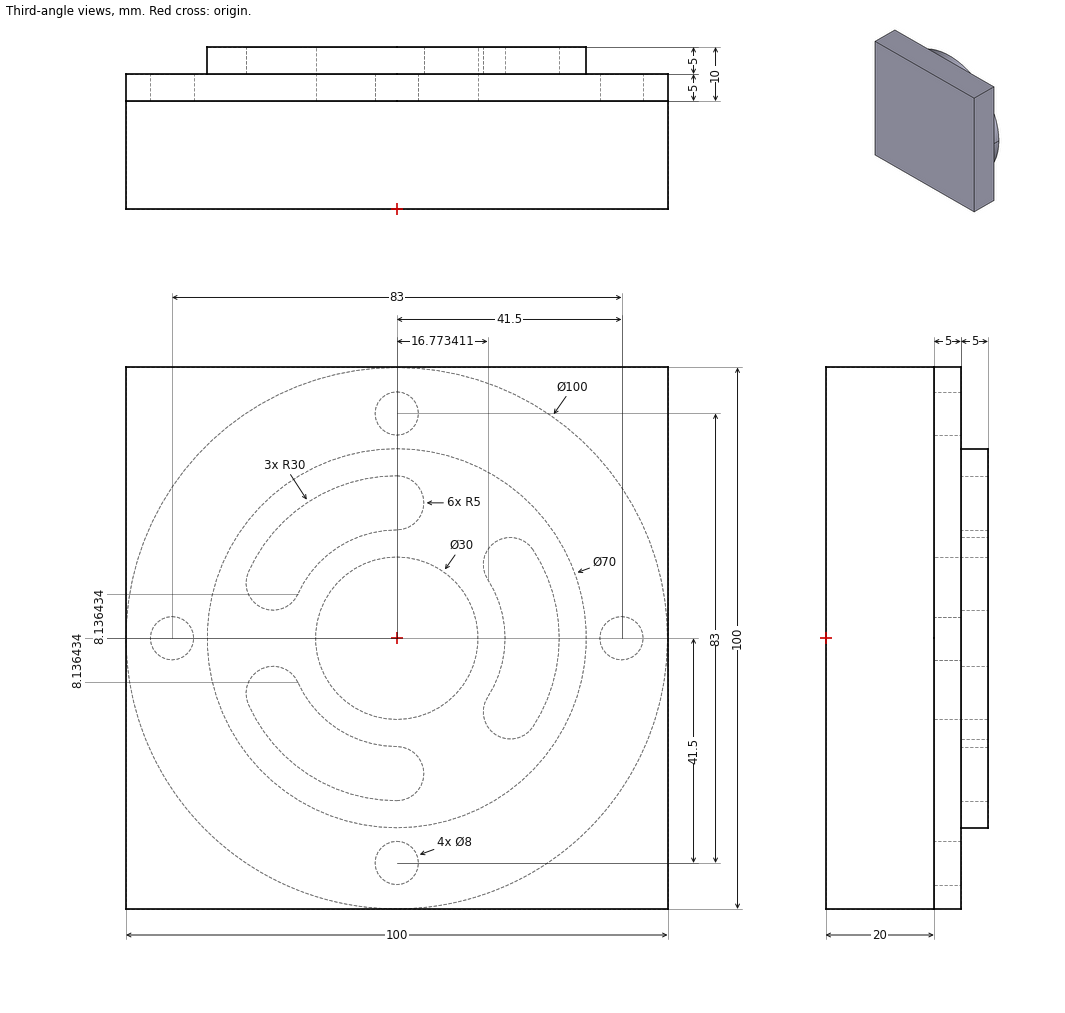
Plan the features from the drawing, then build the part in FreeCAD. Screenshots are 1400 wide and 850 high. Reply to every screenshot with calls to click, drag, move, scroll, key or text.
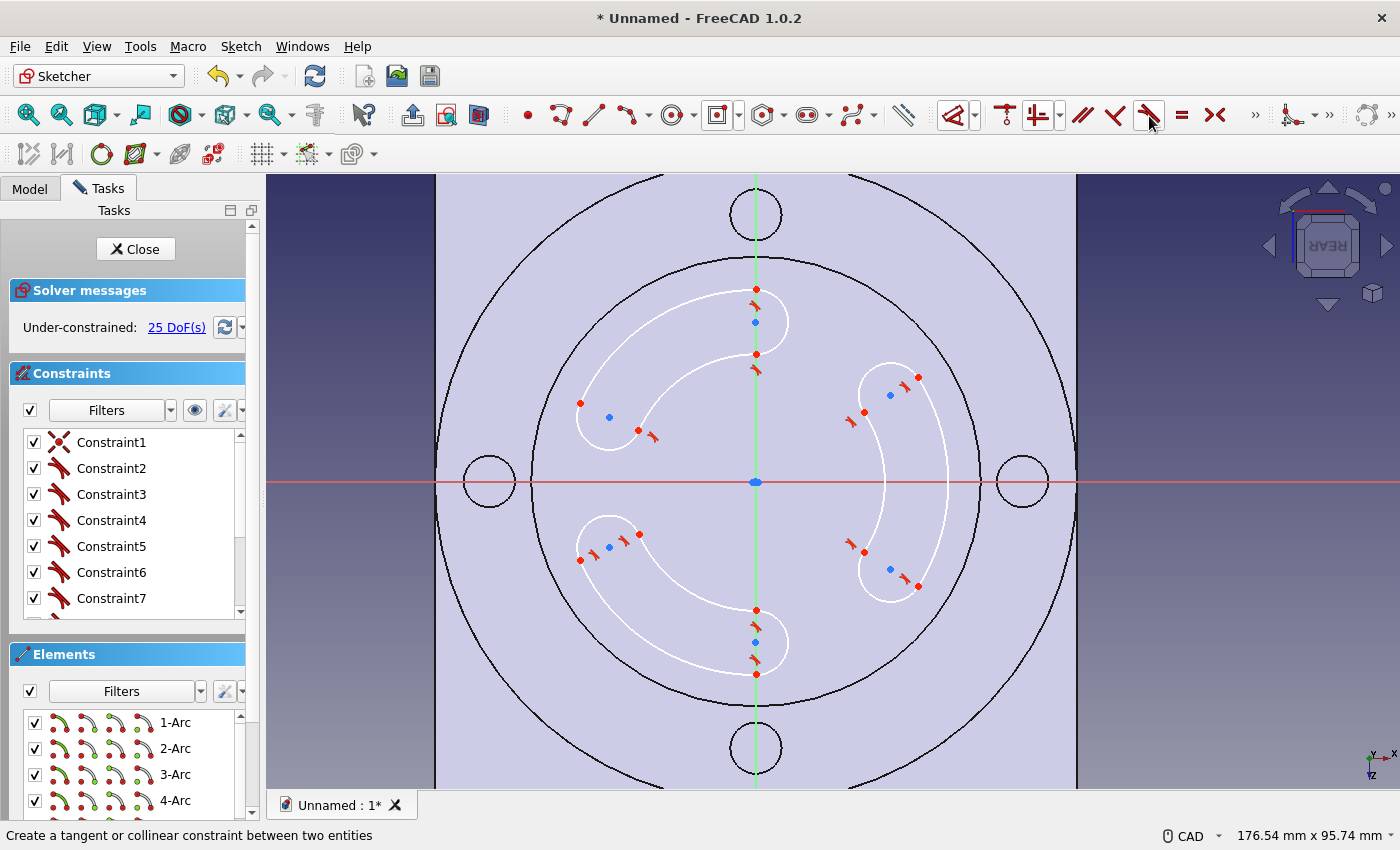
click(691, 301)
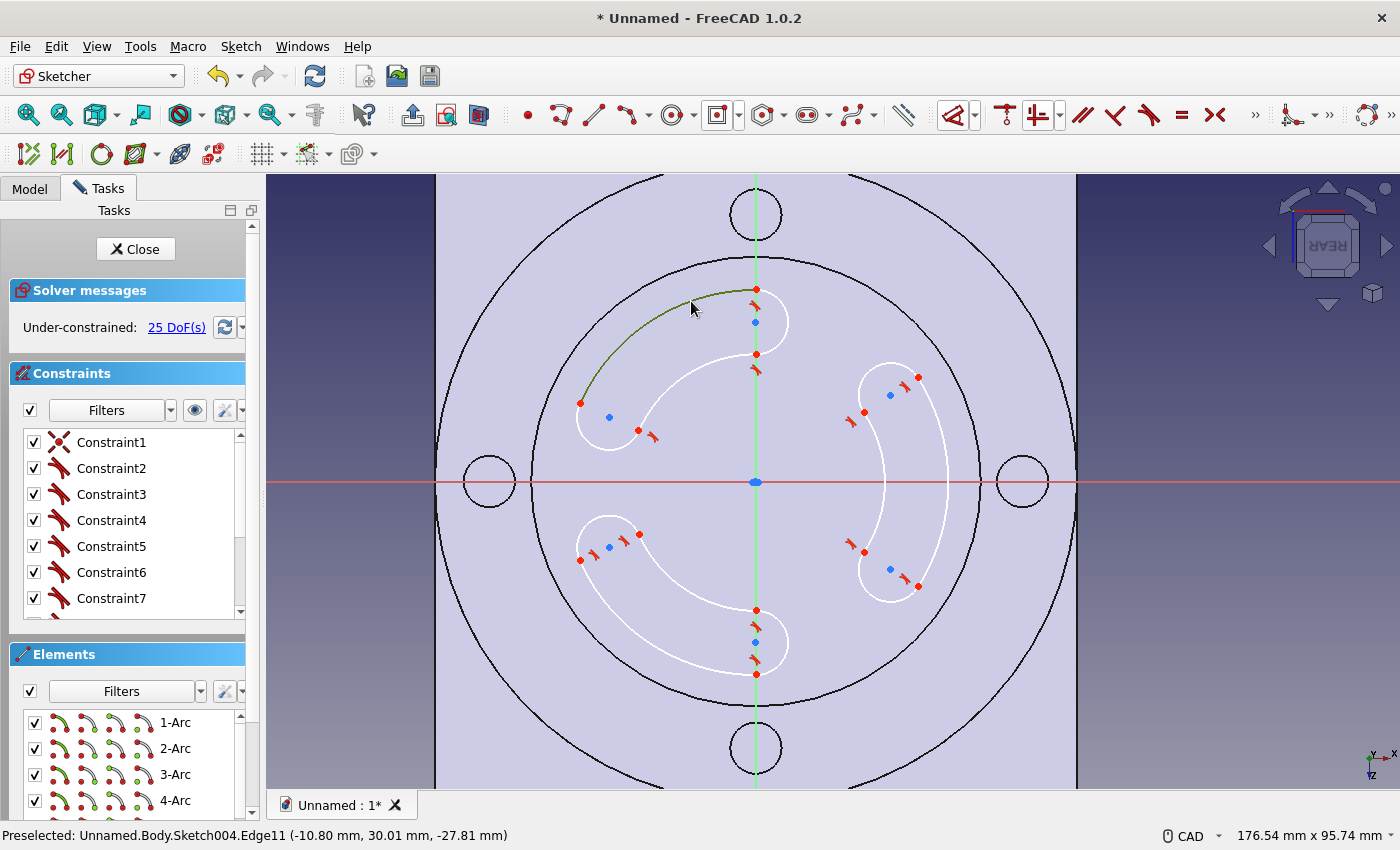
click(581, 434)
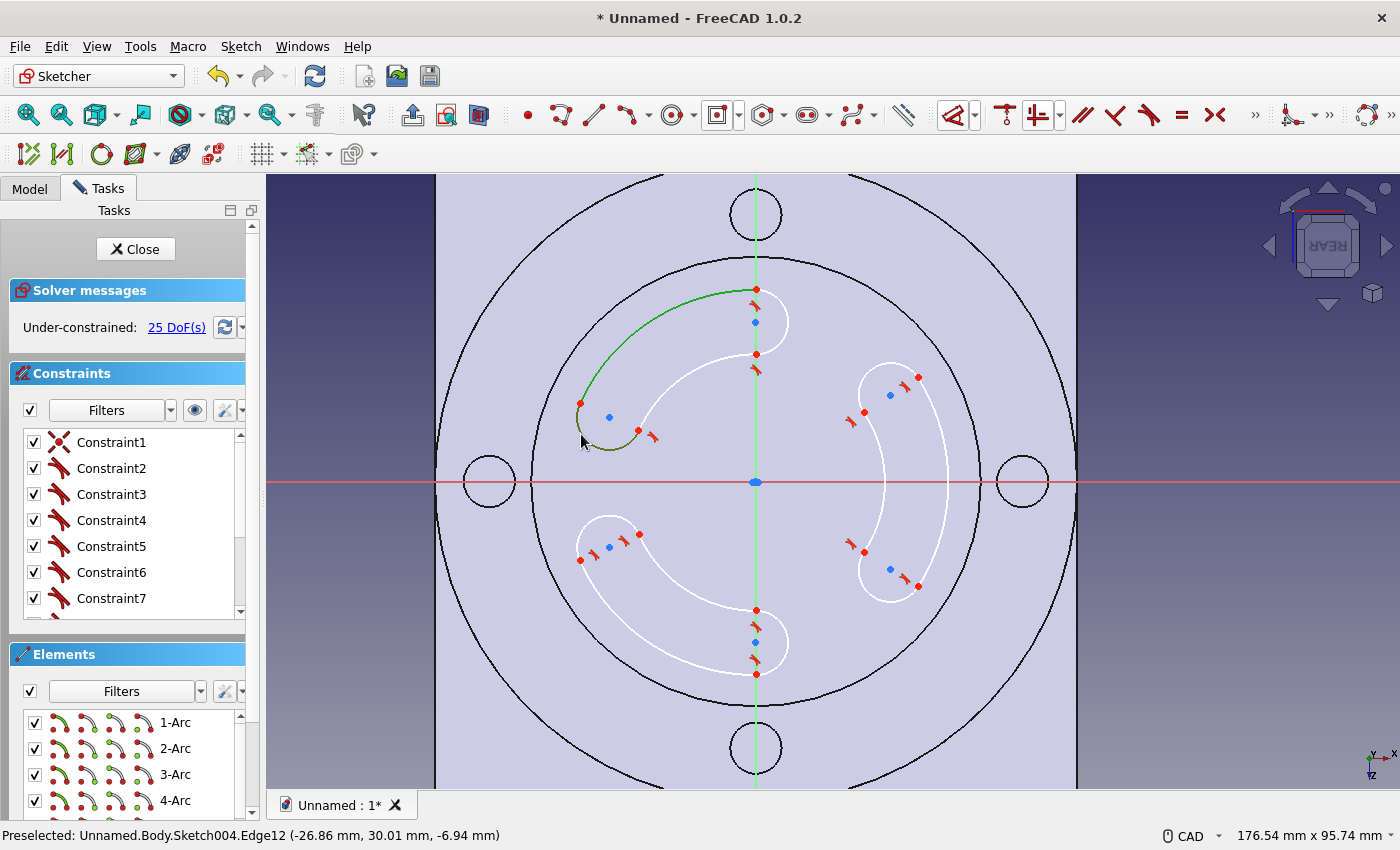
click(1149, 116)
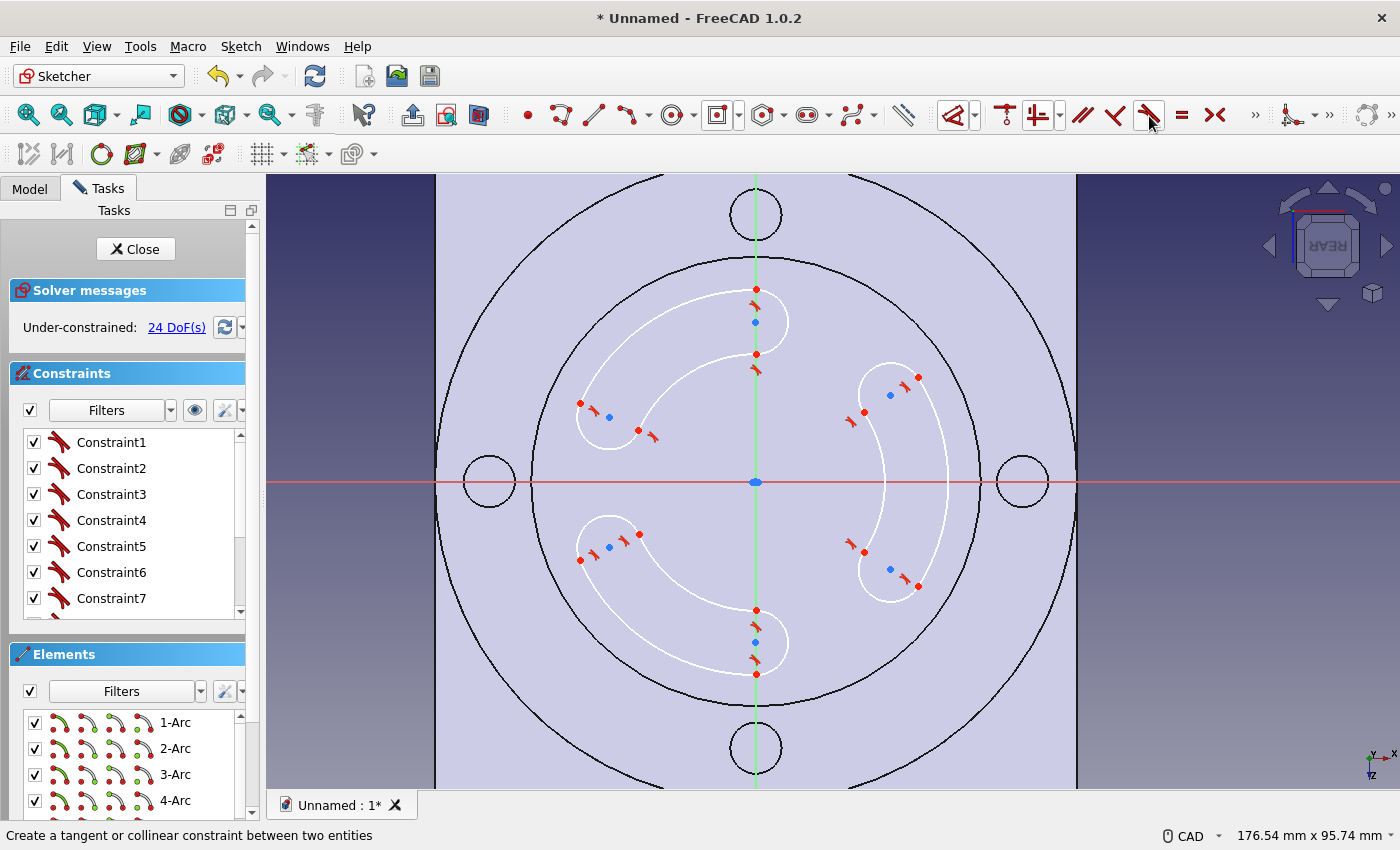
click(617, 616)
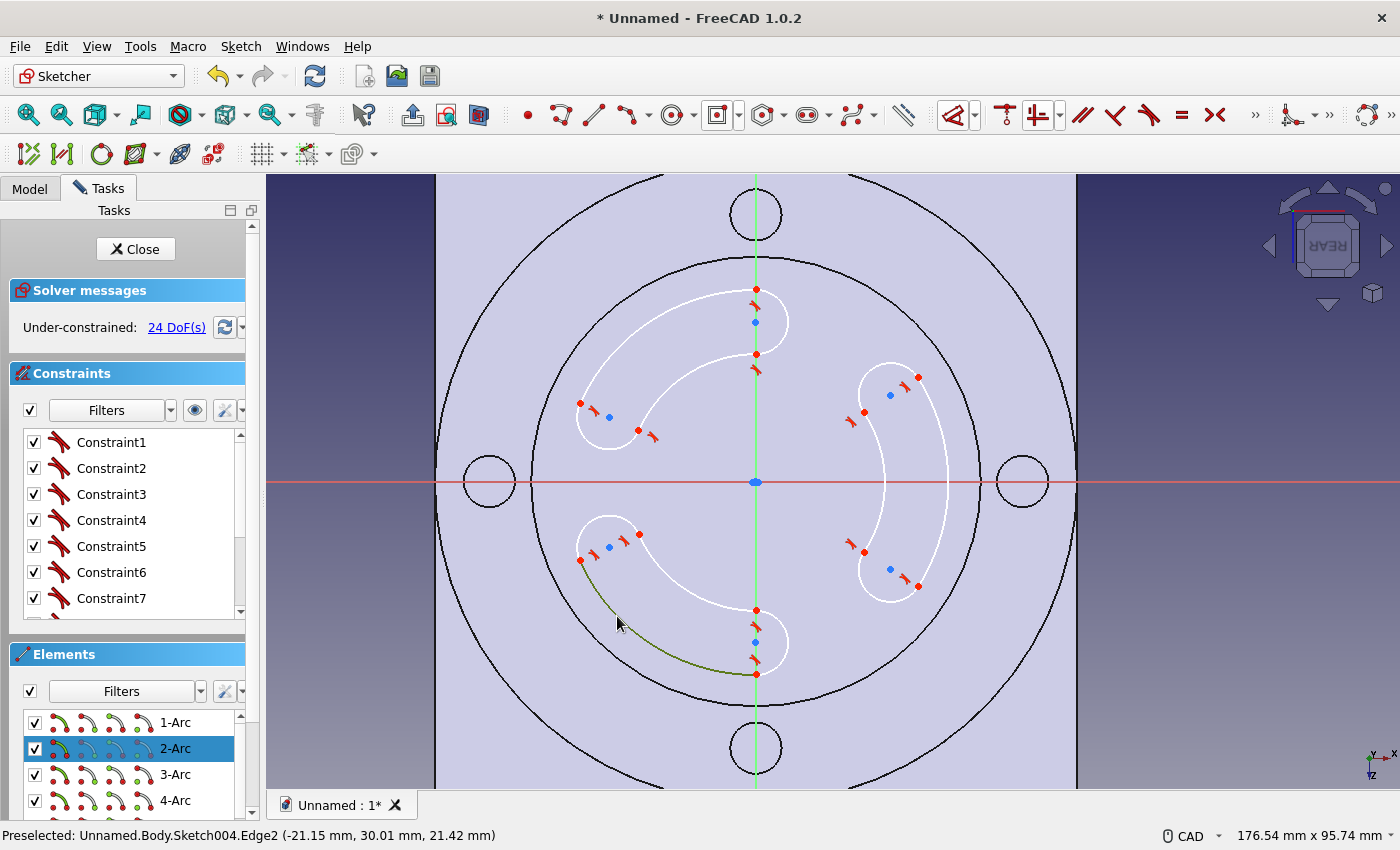
click(664, 571)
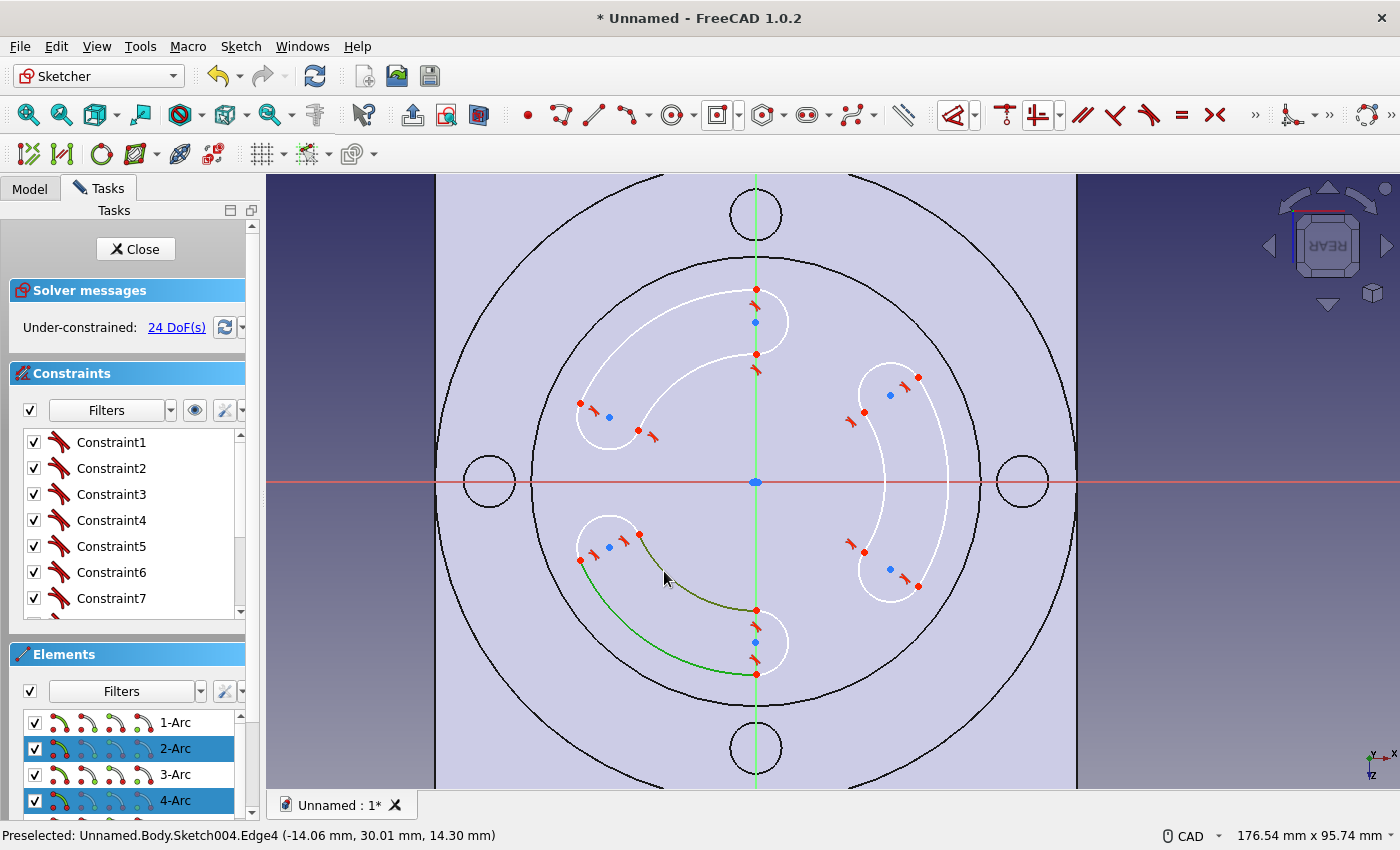
click(1005, 116)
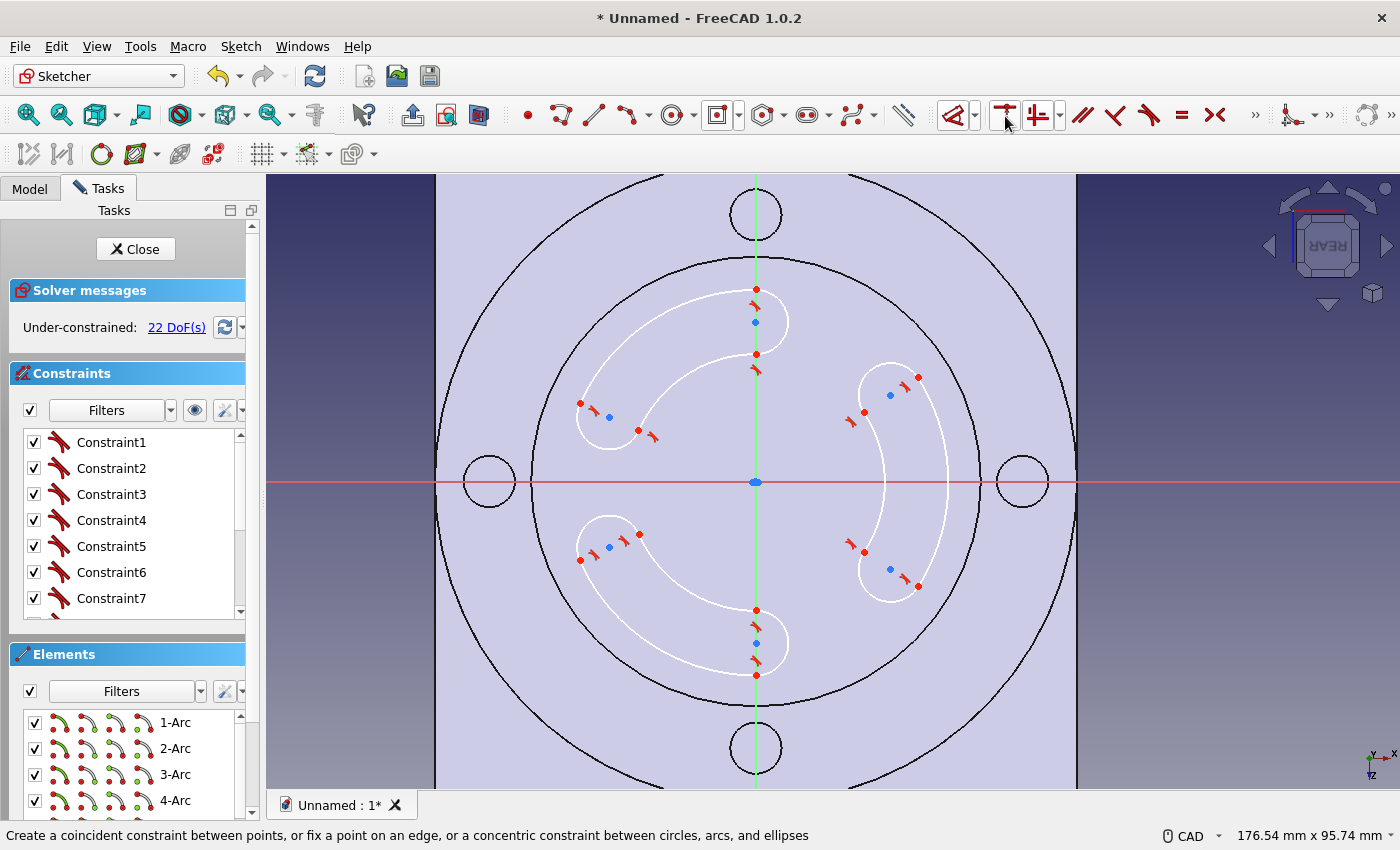
click(617, 616)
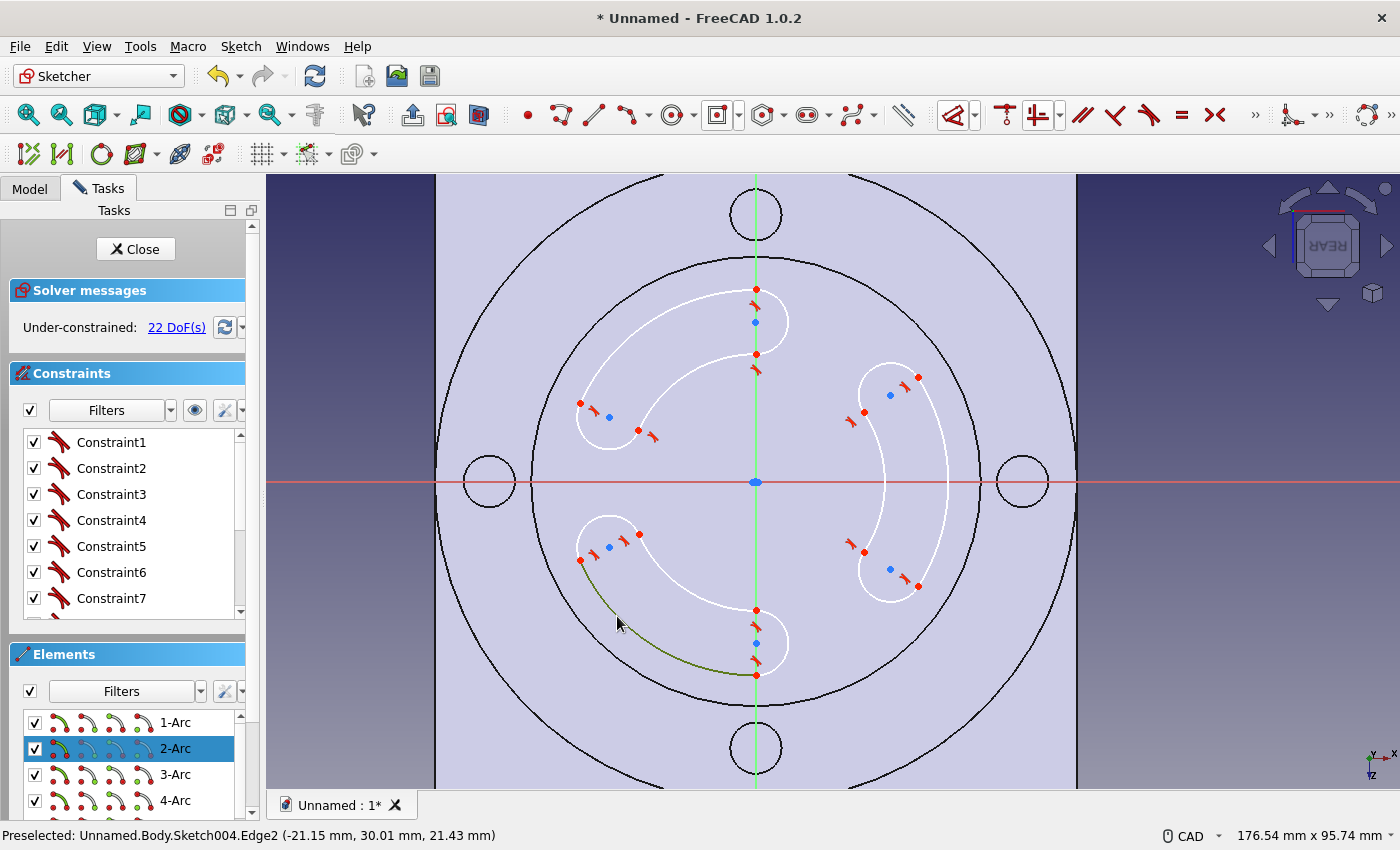
click(881, 512)